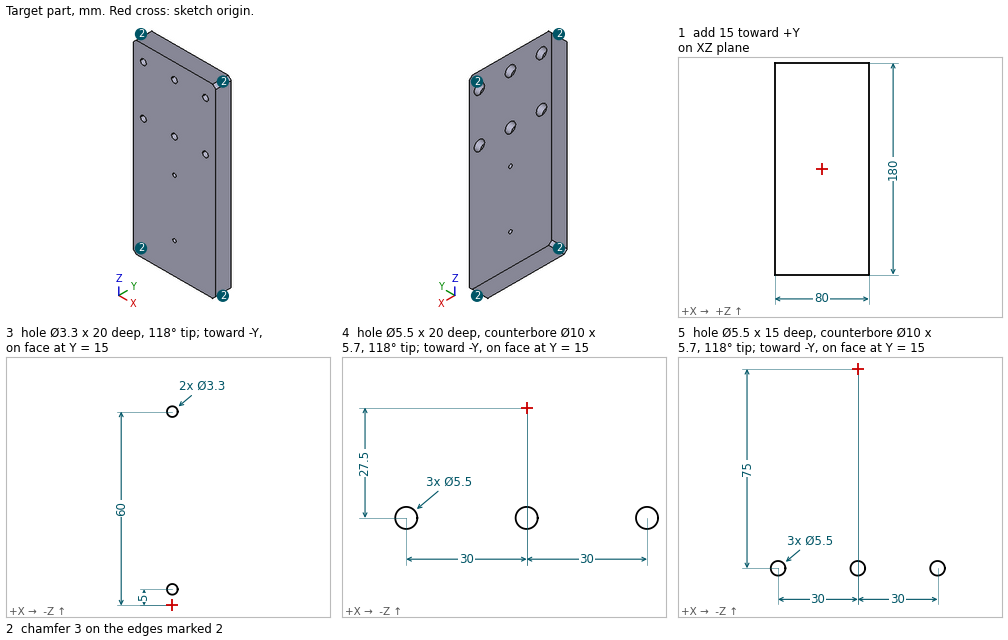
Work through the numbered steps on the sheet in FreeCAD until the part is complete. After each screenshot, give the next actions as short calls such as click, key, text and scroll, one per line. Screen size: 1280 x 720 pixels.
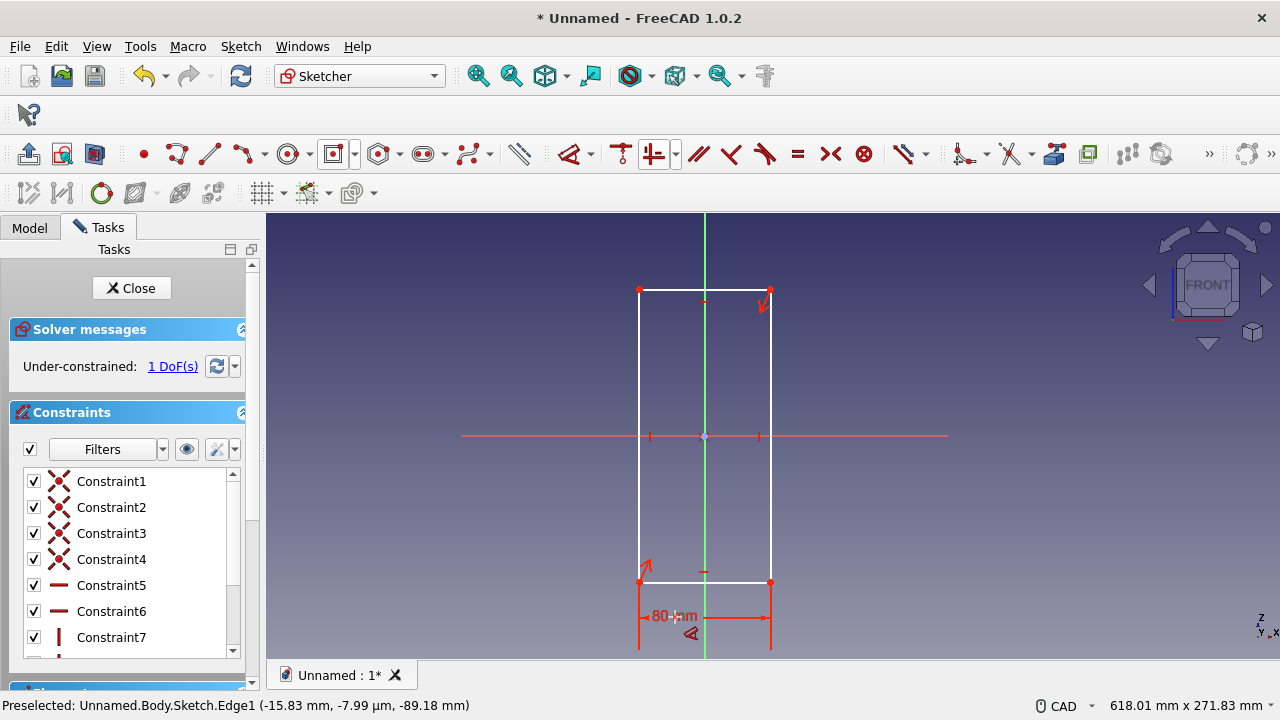
click(771, 495)
click(805, 369)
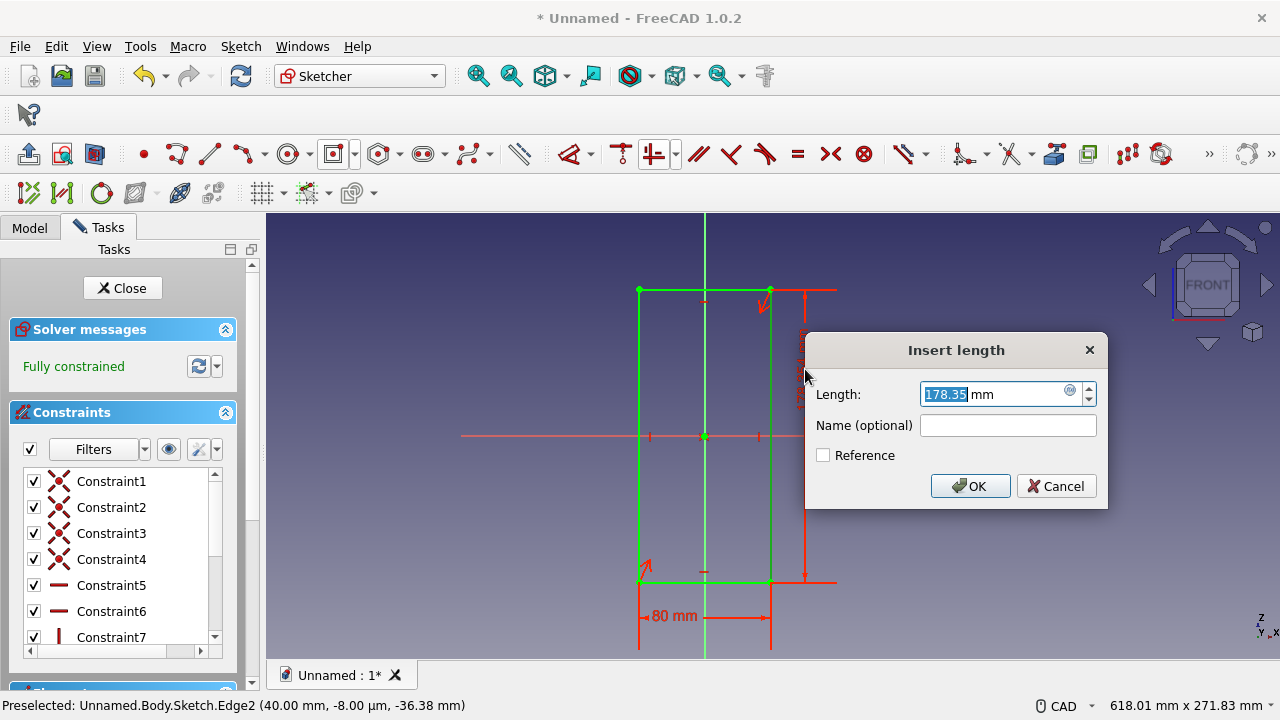
text(180)
key(Return)
key(Escape)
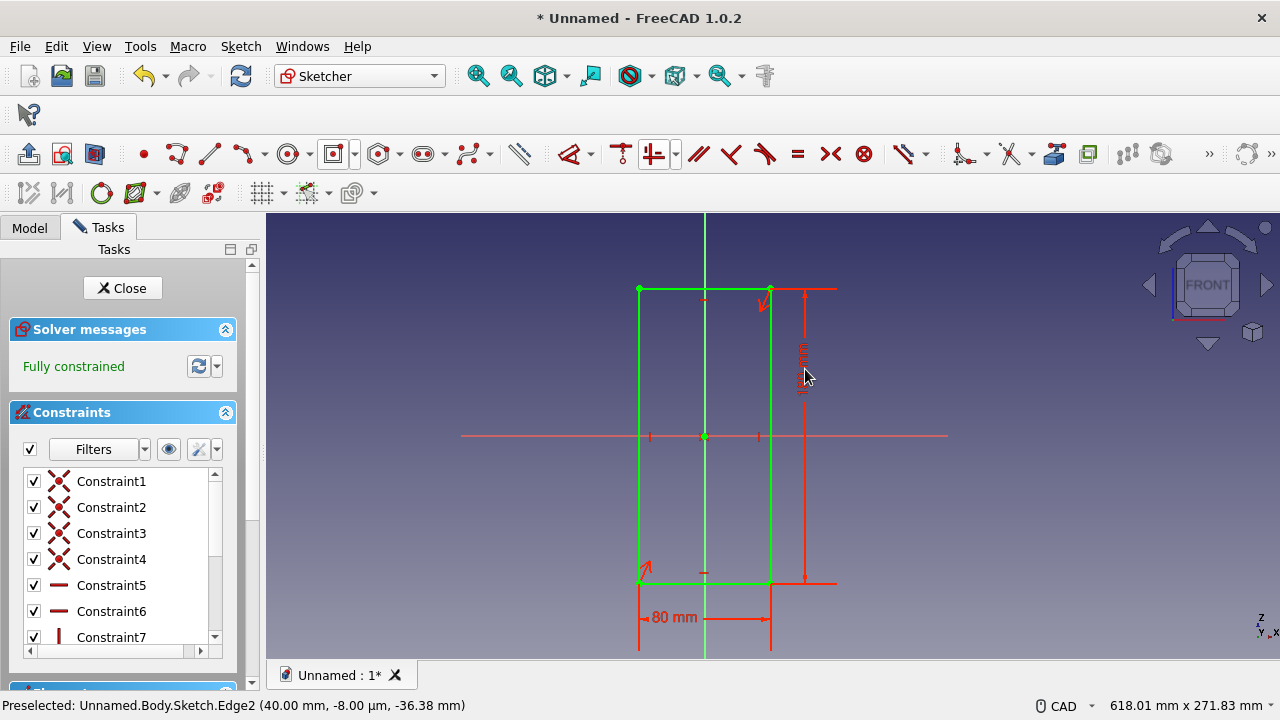
click(123, 288)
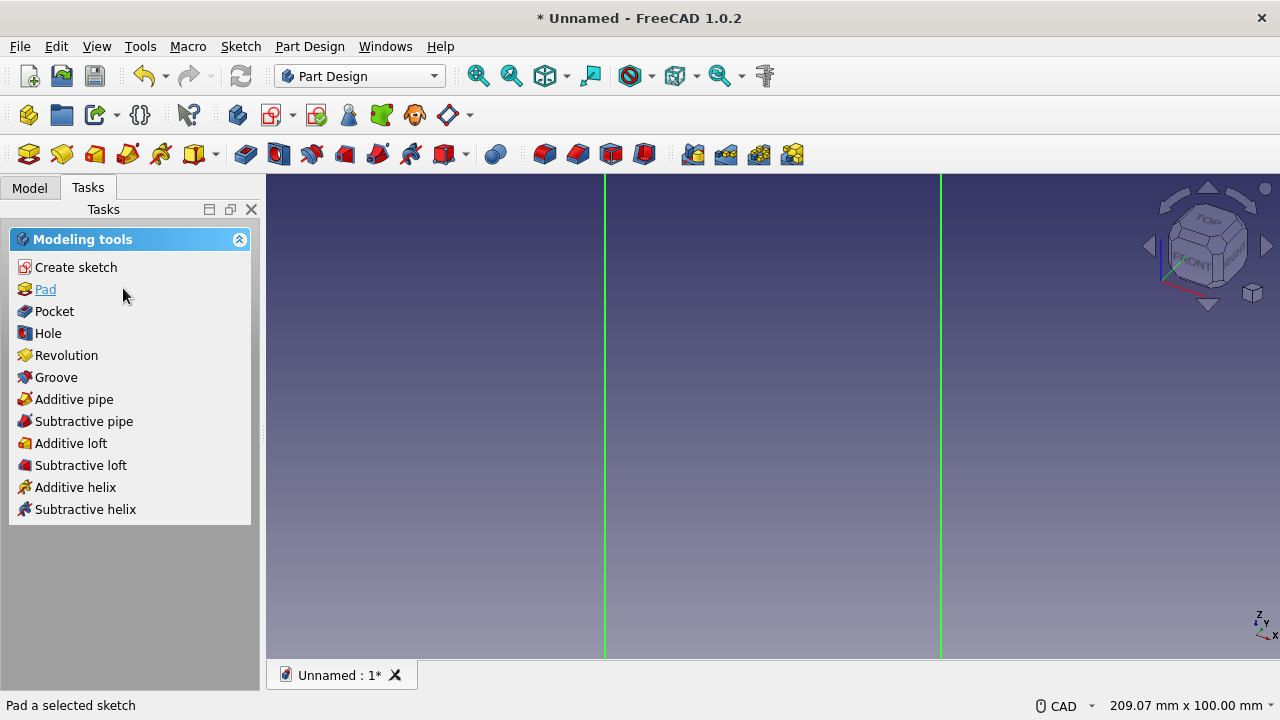
click(29, 154)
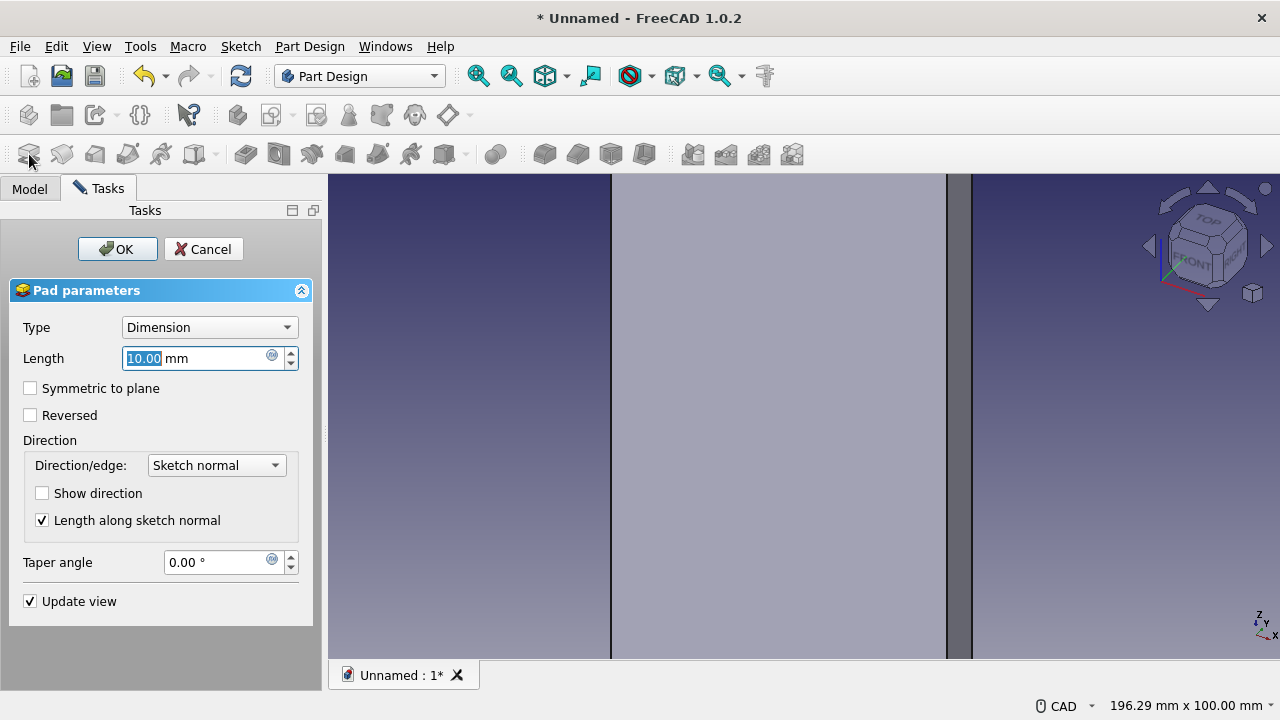
text(15)
key(Tab)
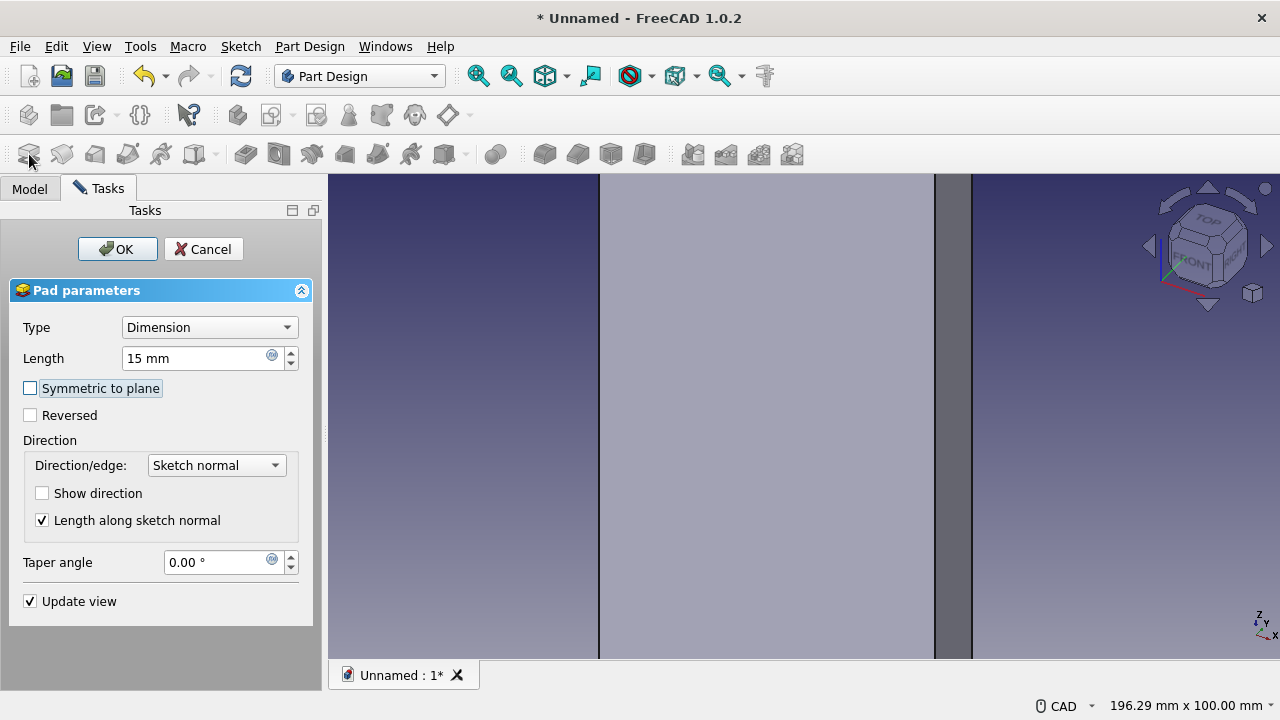
click(31, 415)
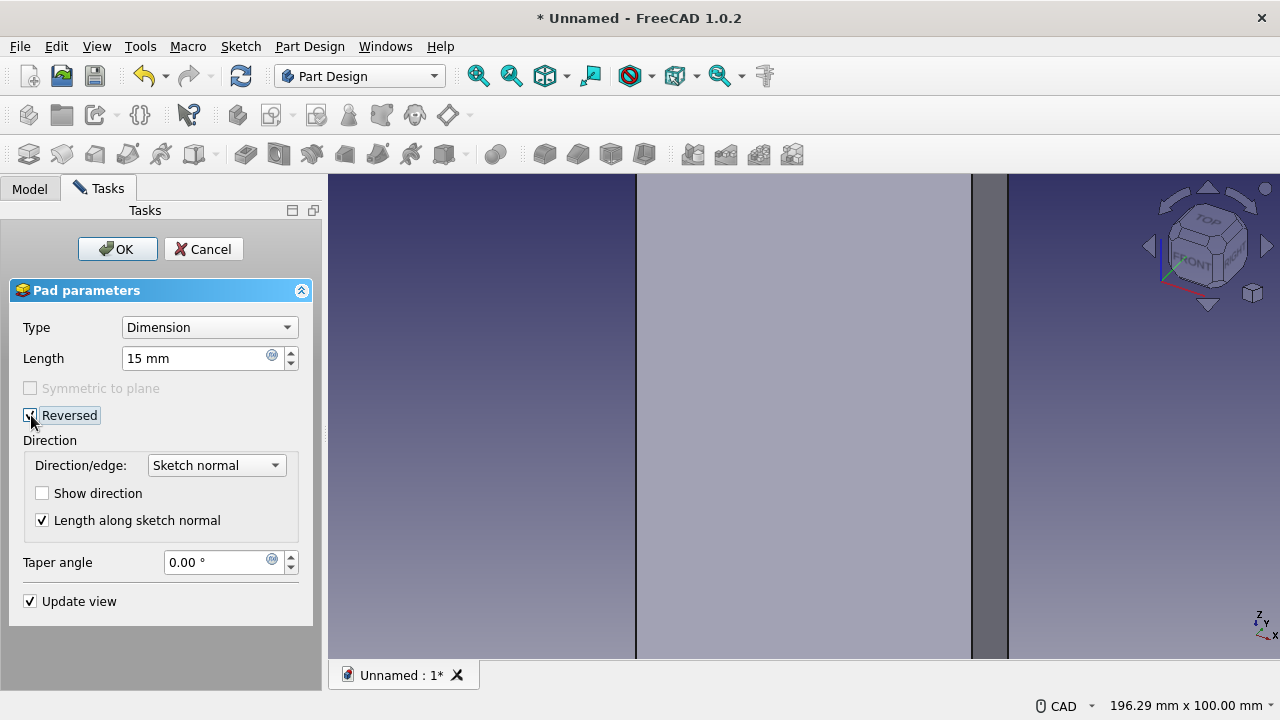
click(118, 249)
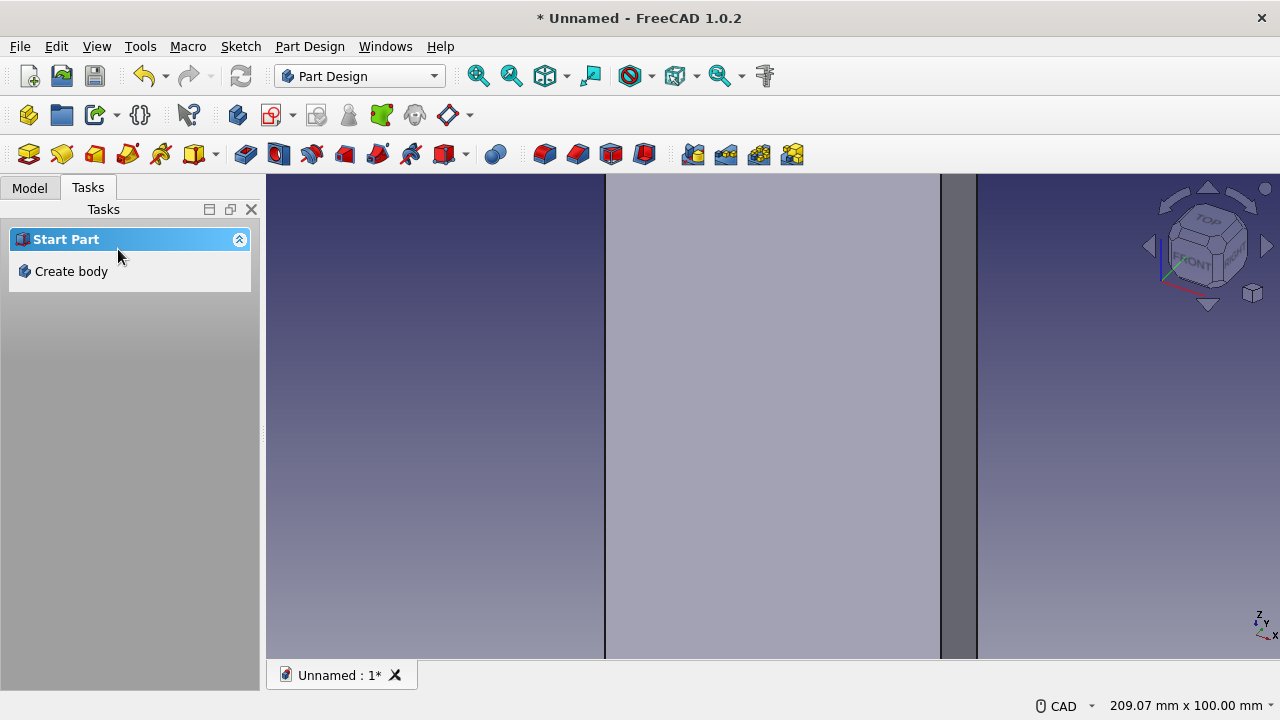
click(479, 76)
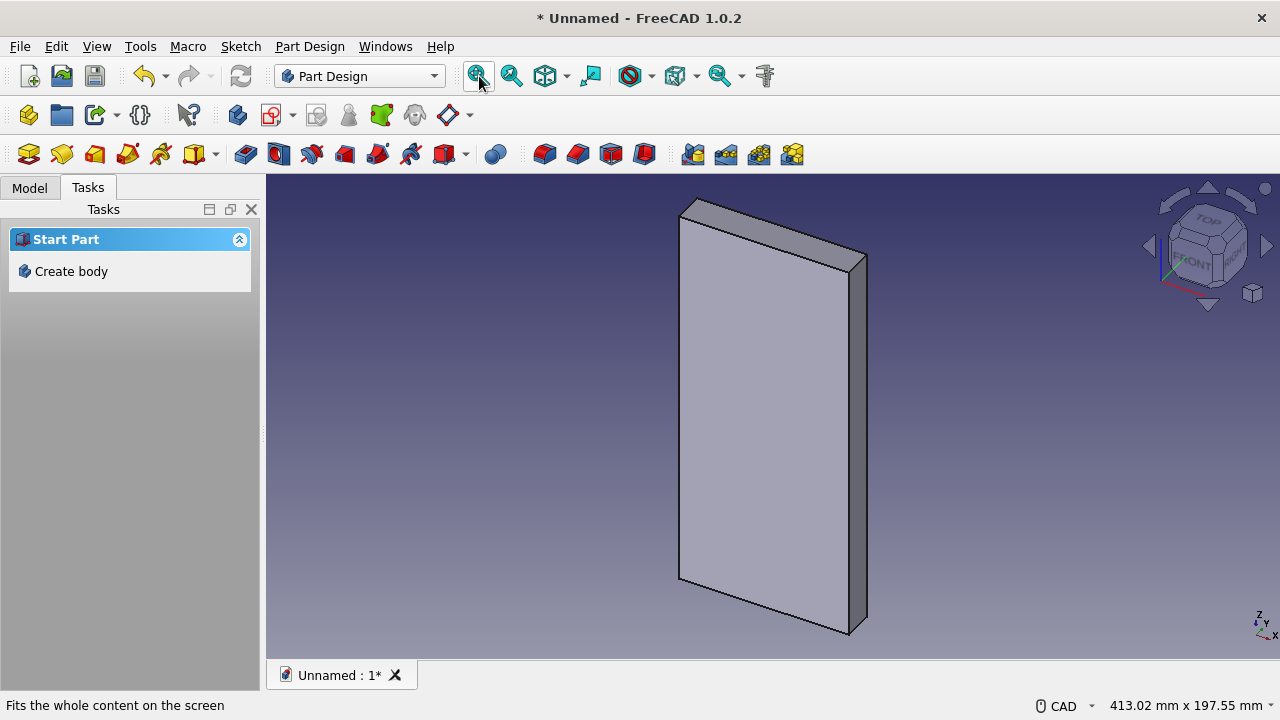
click(858, 263)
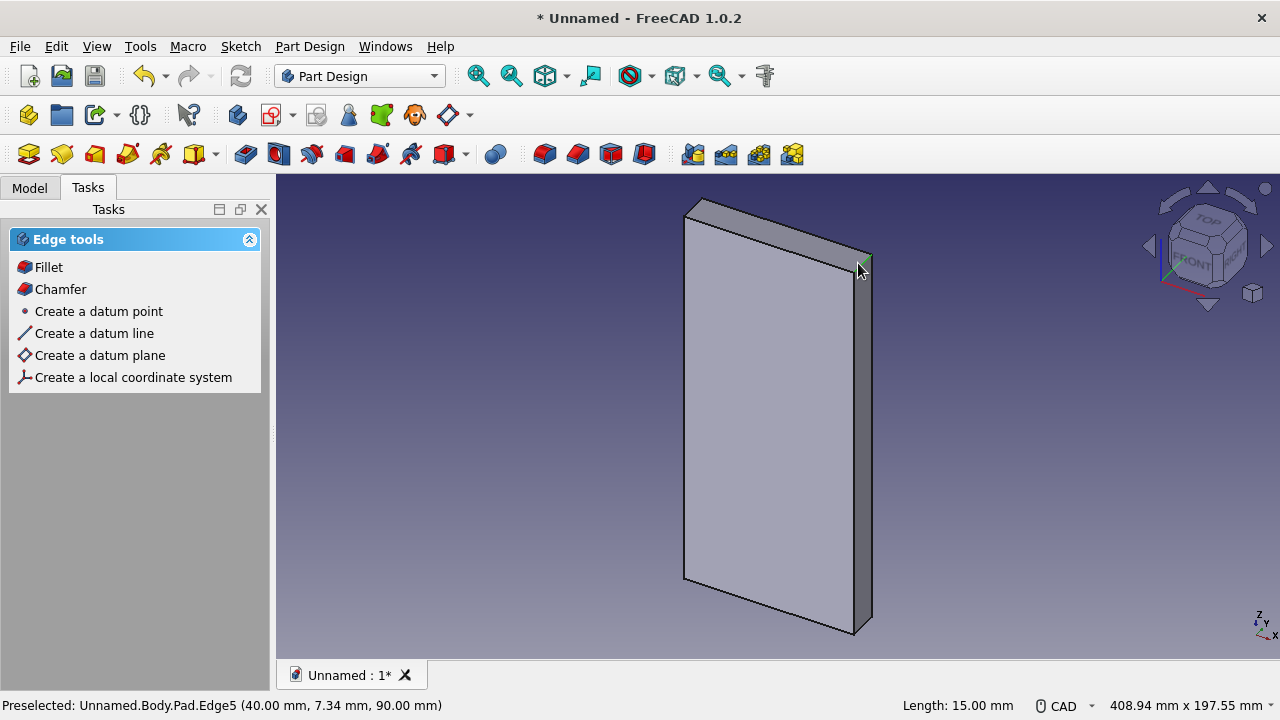
key(0)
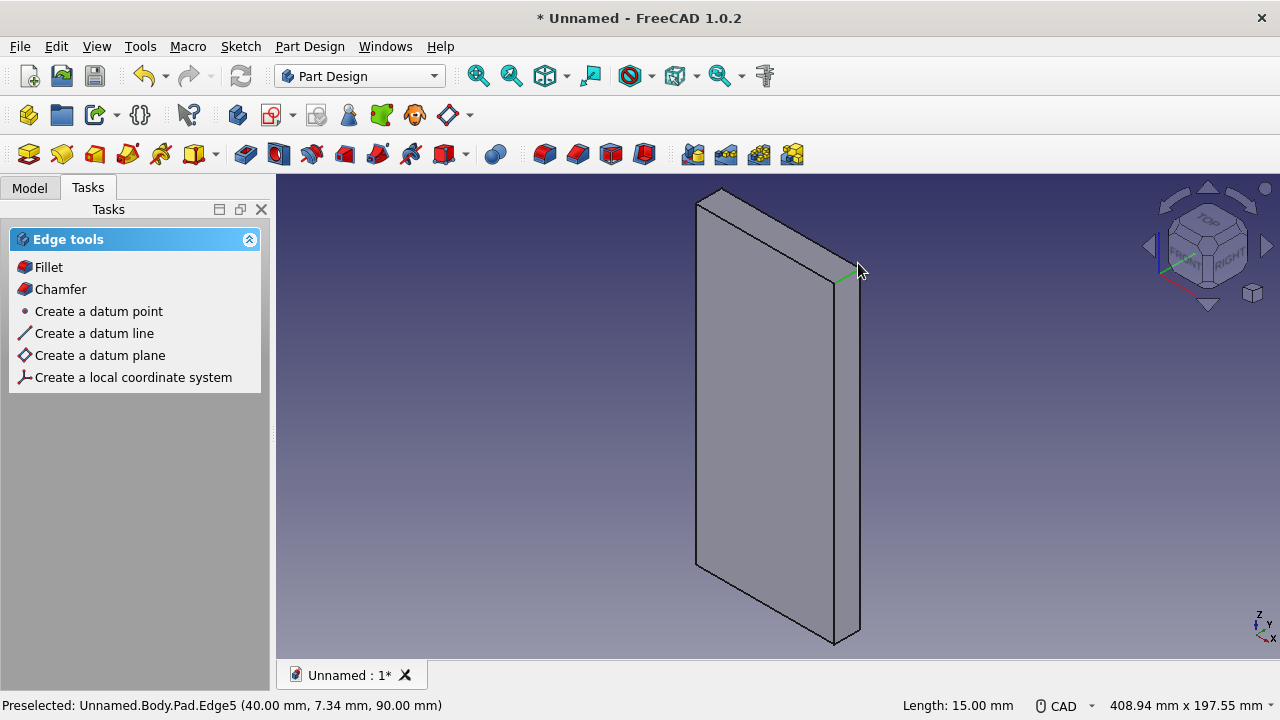
key(2)